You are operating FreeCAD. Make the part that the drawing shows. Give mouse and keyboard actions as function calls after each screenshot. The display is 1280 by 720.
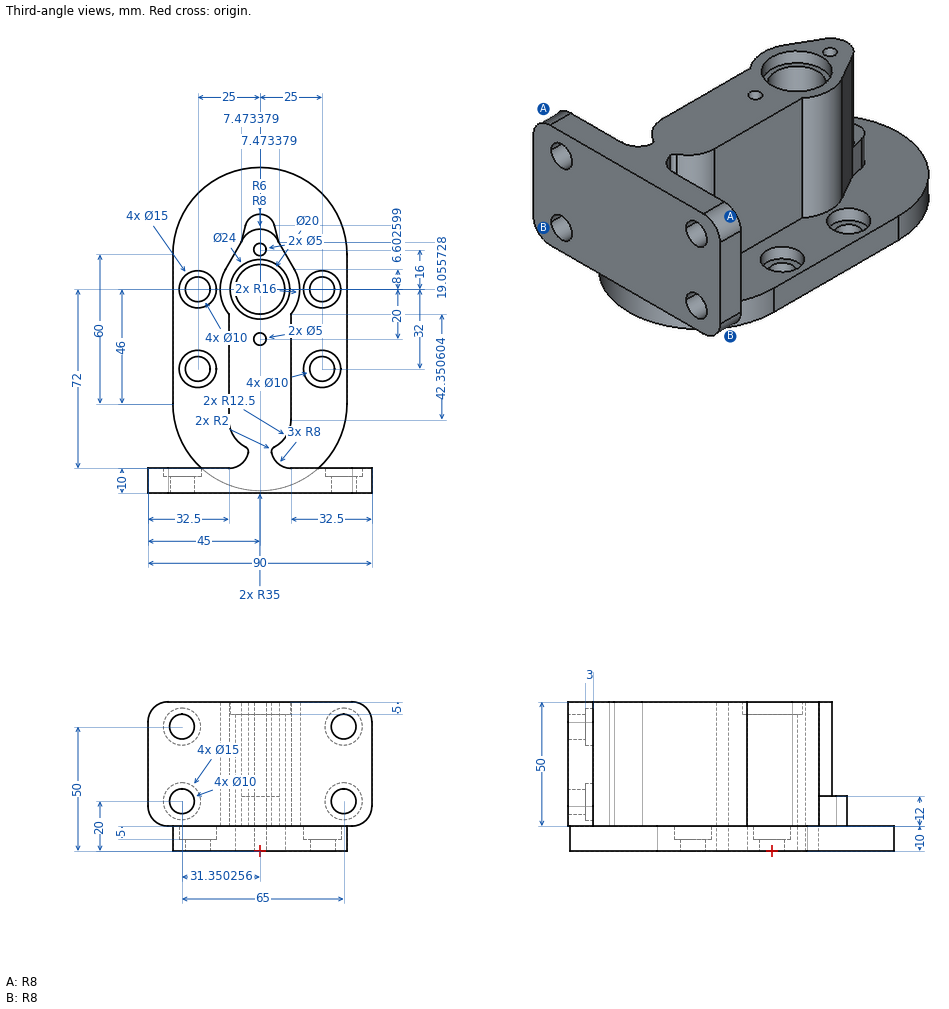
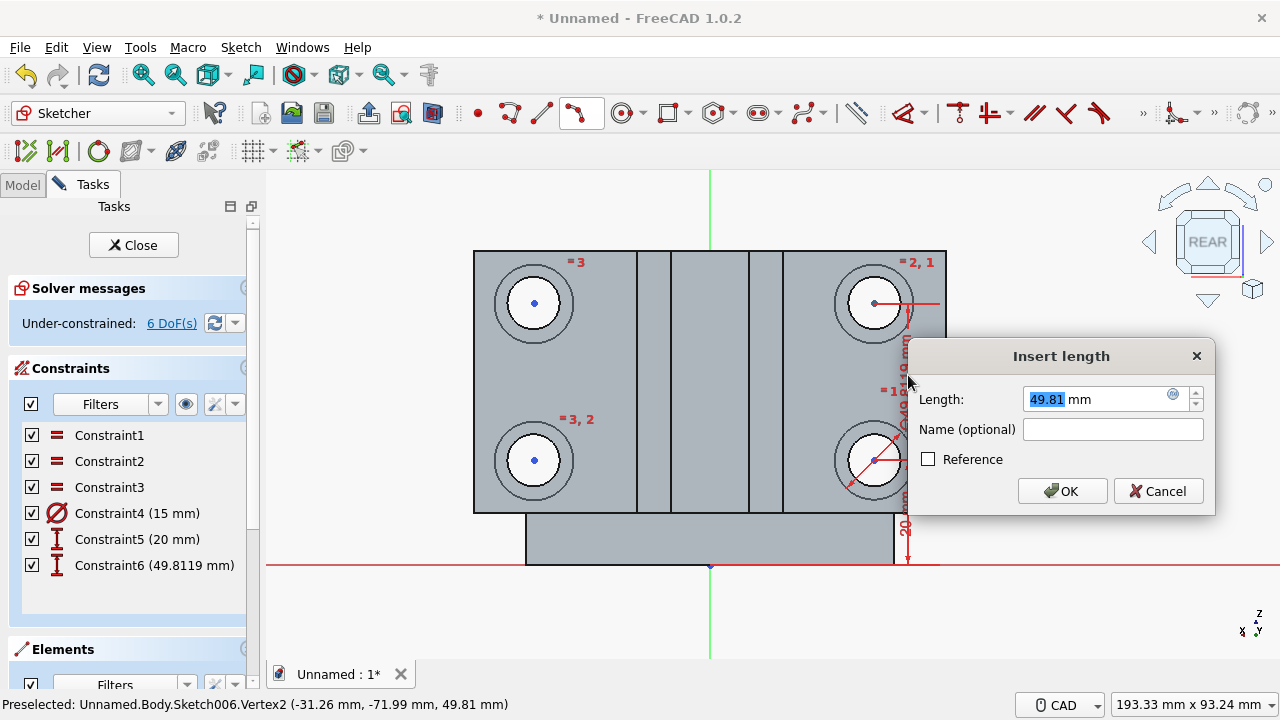
text(50)
key(Return)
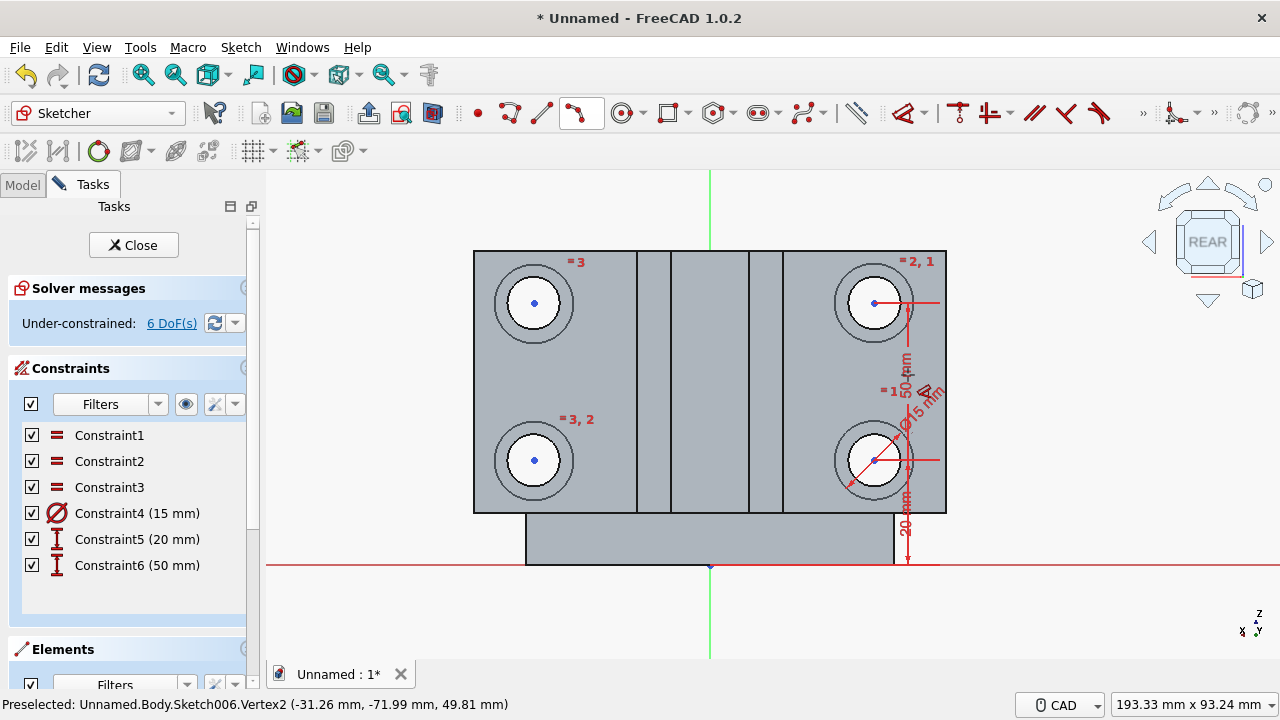
click(534, 461)
click(500, 513)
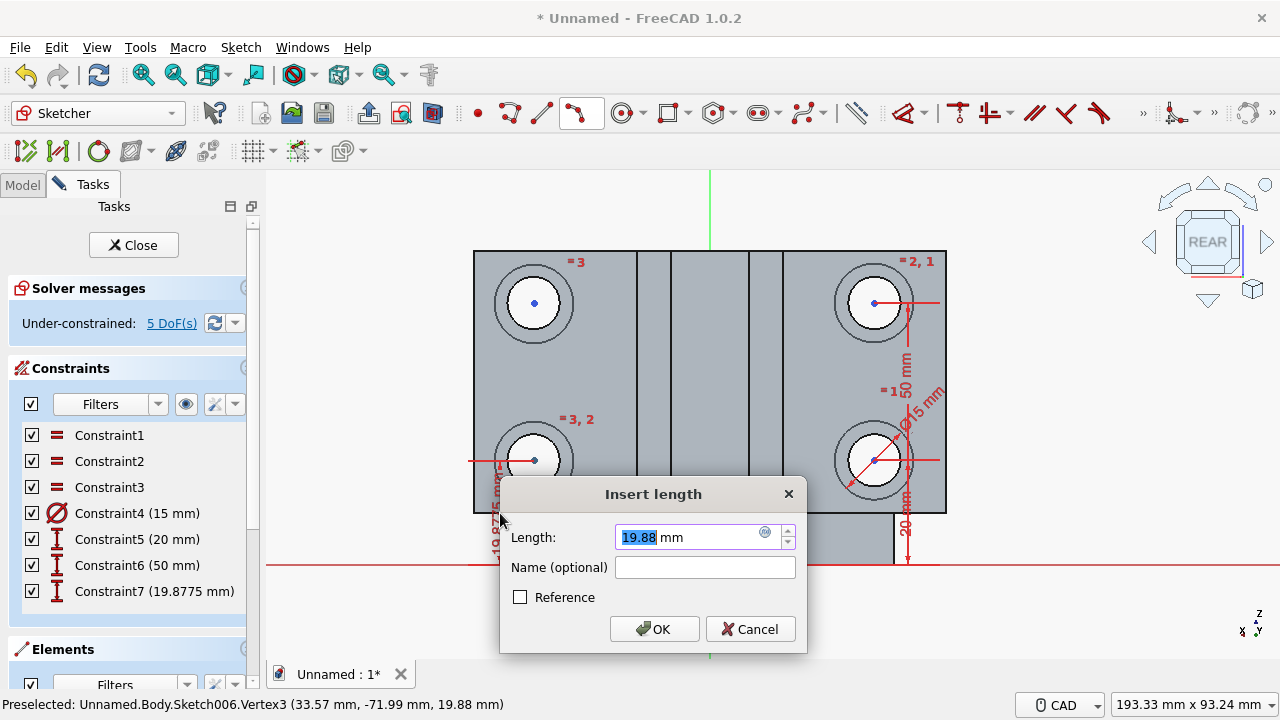
text(20)
key(Return)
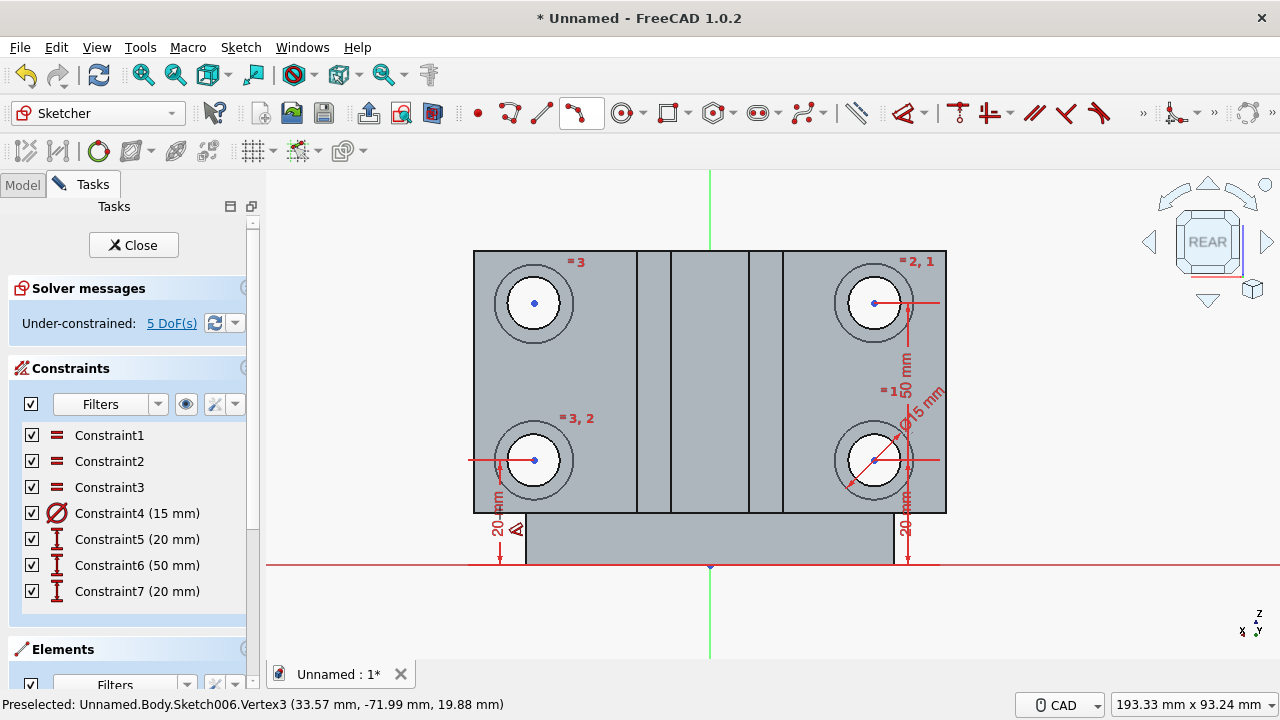
click(534, 304)
click(500, 375)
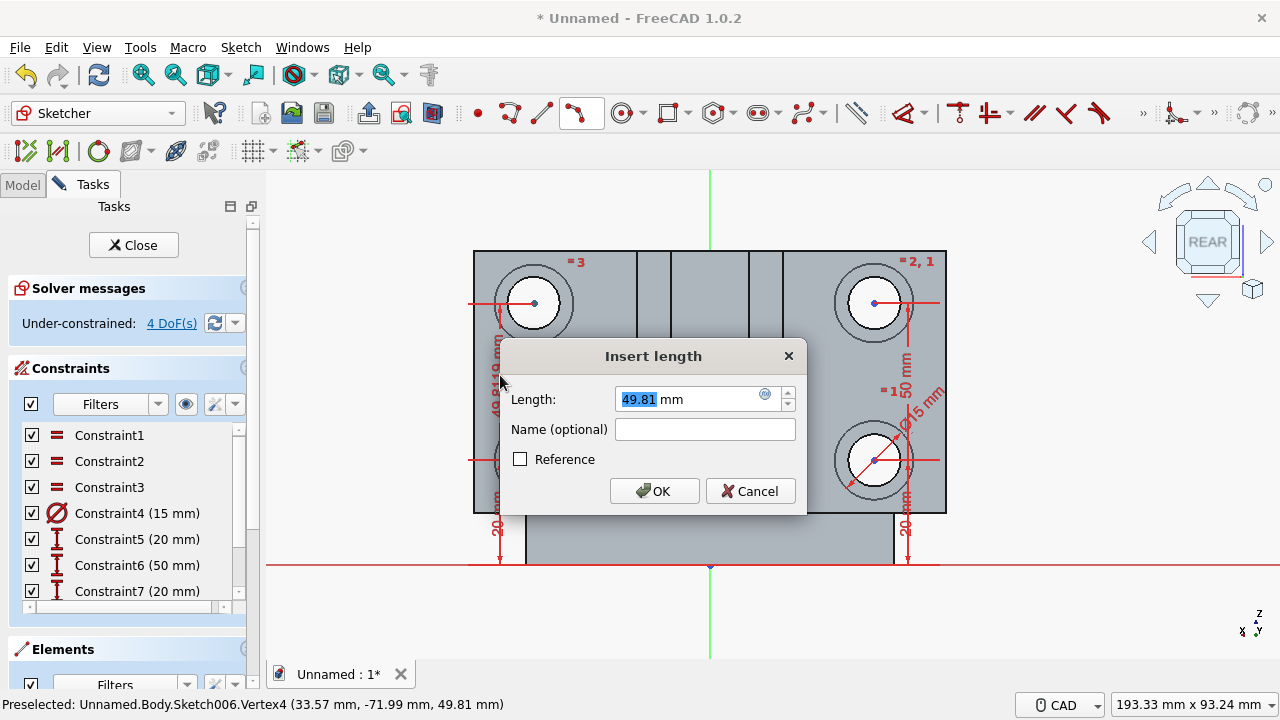
text(50)
key(Return)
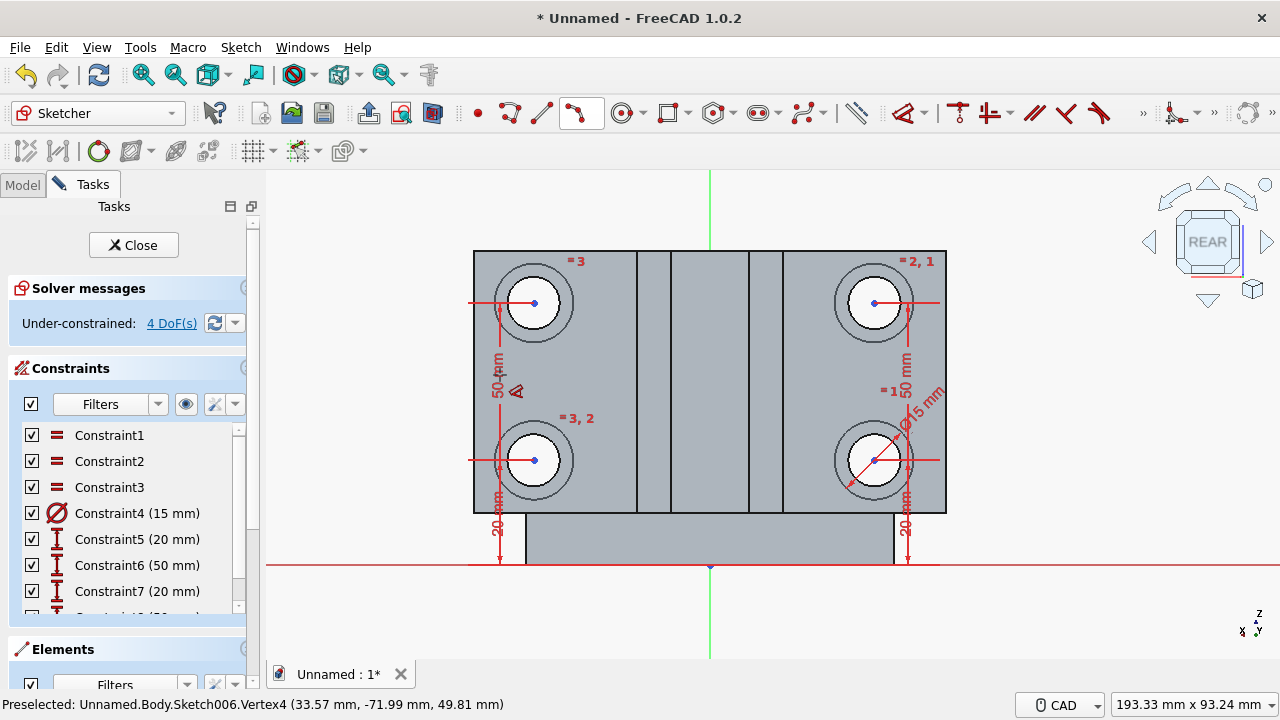
click(874, 460)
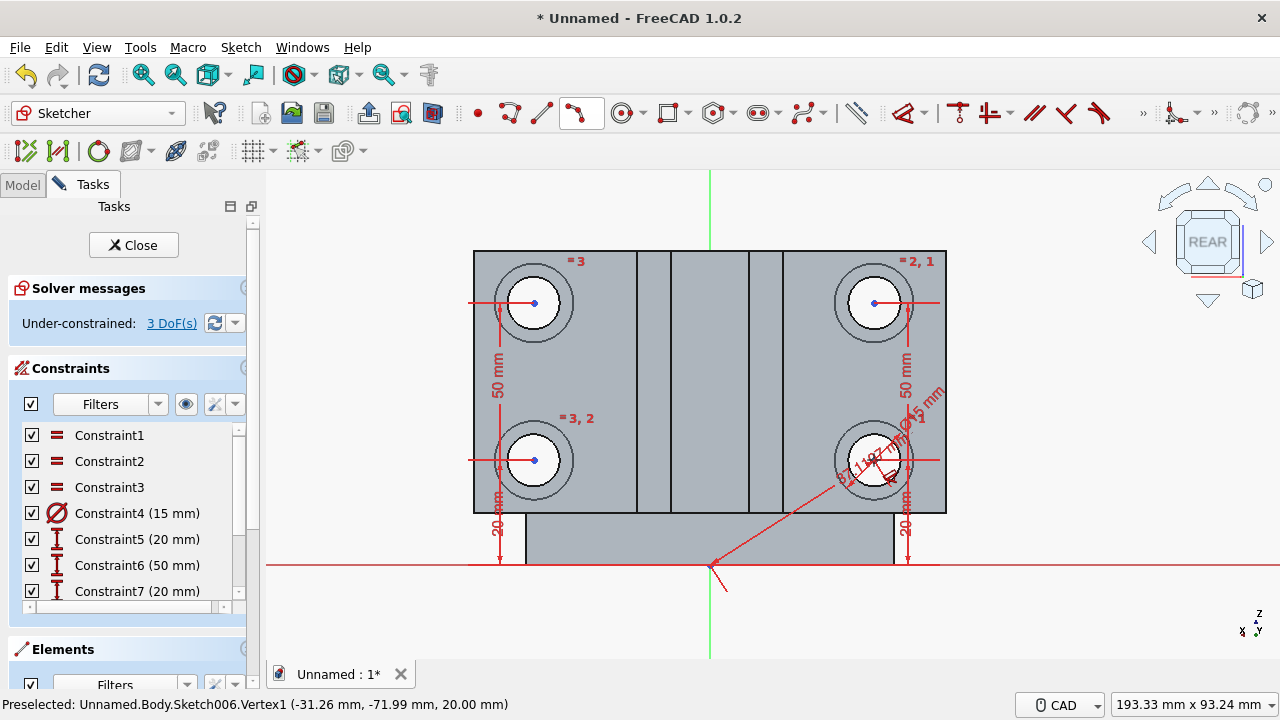
click(534, 460)
click(626, 494)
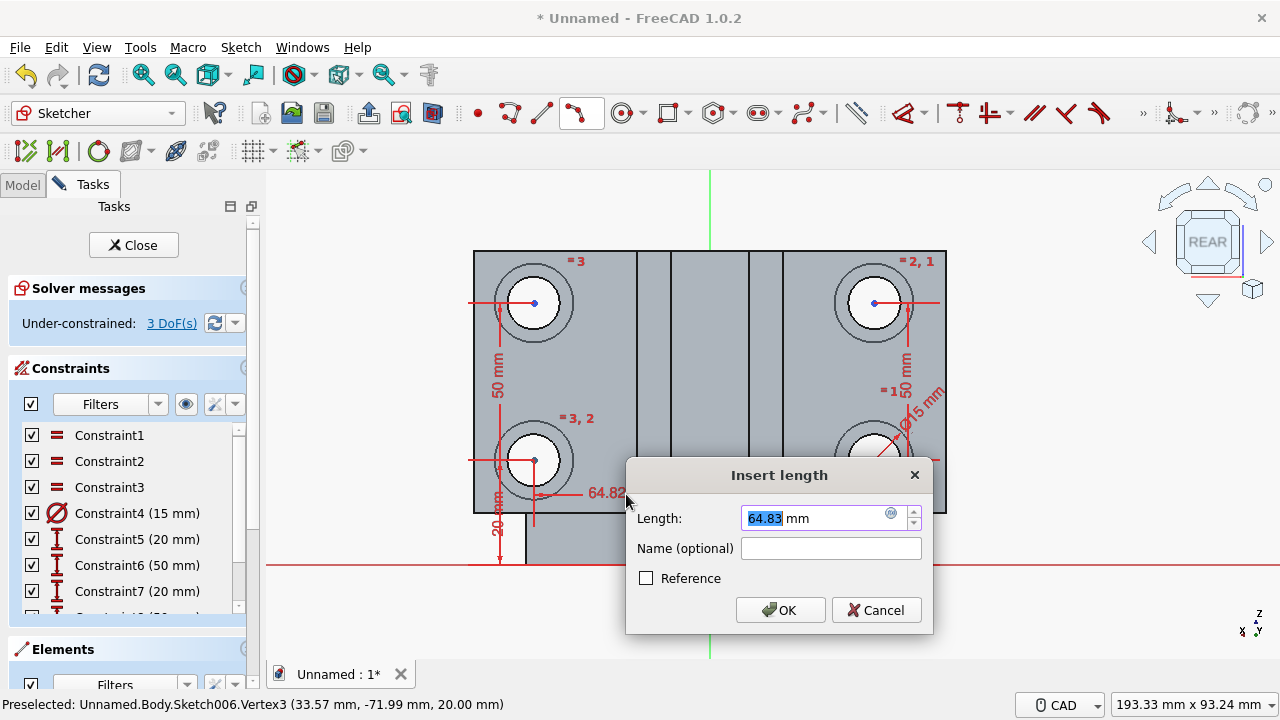
text(65)
key(Return)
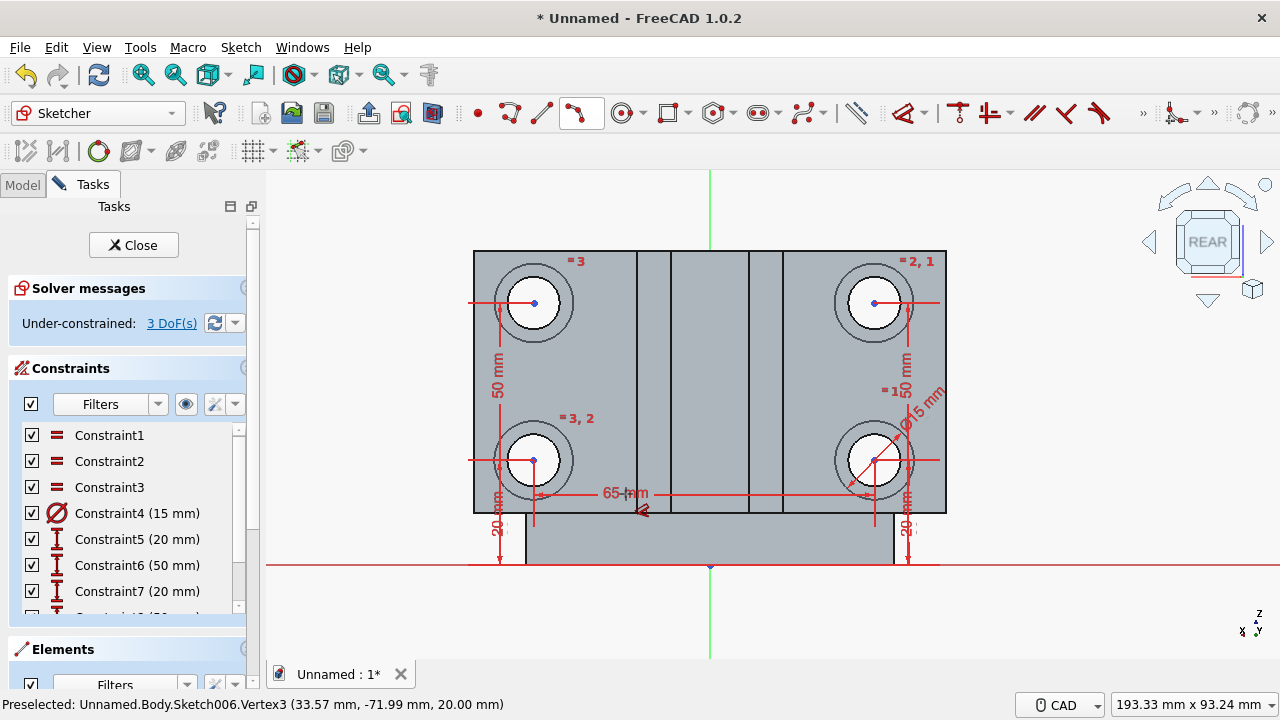
click(874, 303)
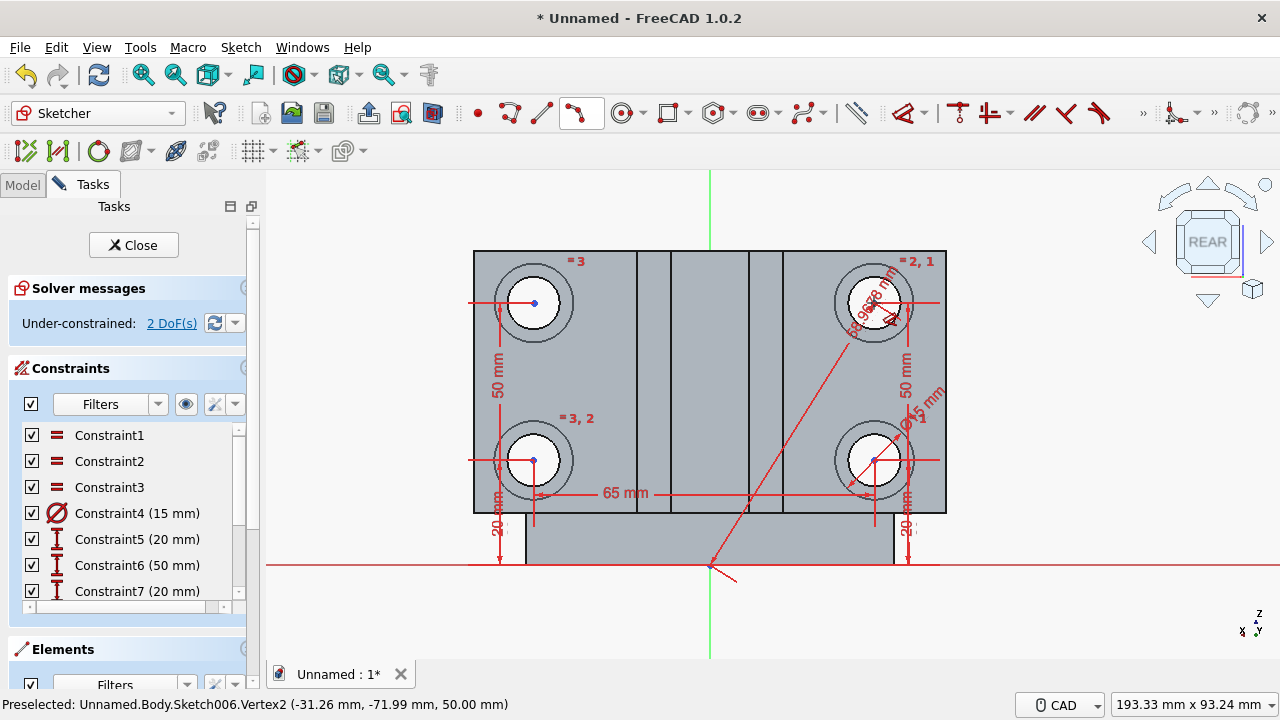
click(534, 460)
click(626, 269)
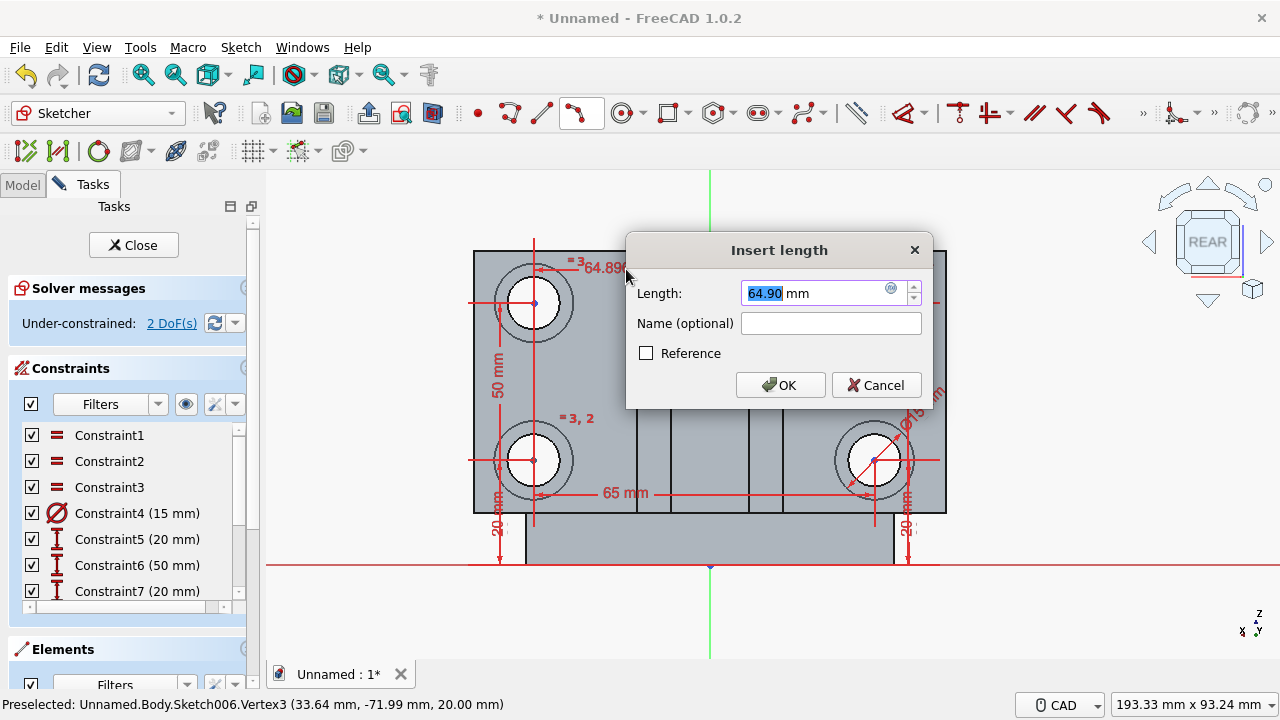
text(65)
key(Return)